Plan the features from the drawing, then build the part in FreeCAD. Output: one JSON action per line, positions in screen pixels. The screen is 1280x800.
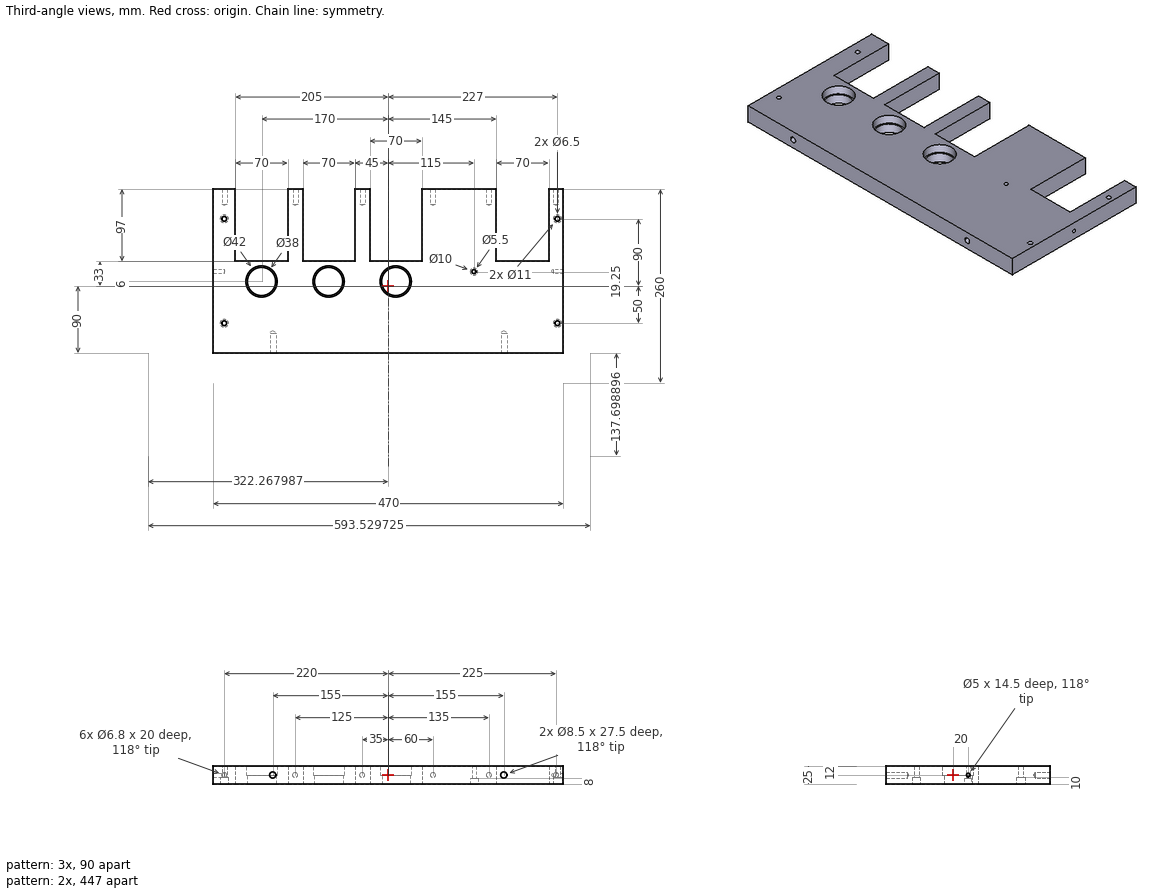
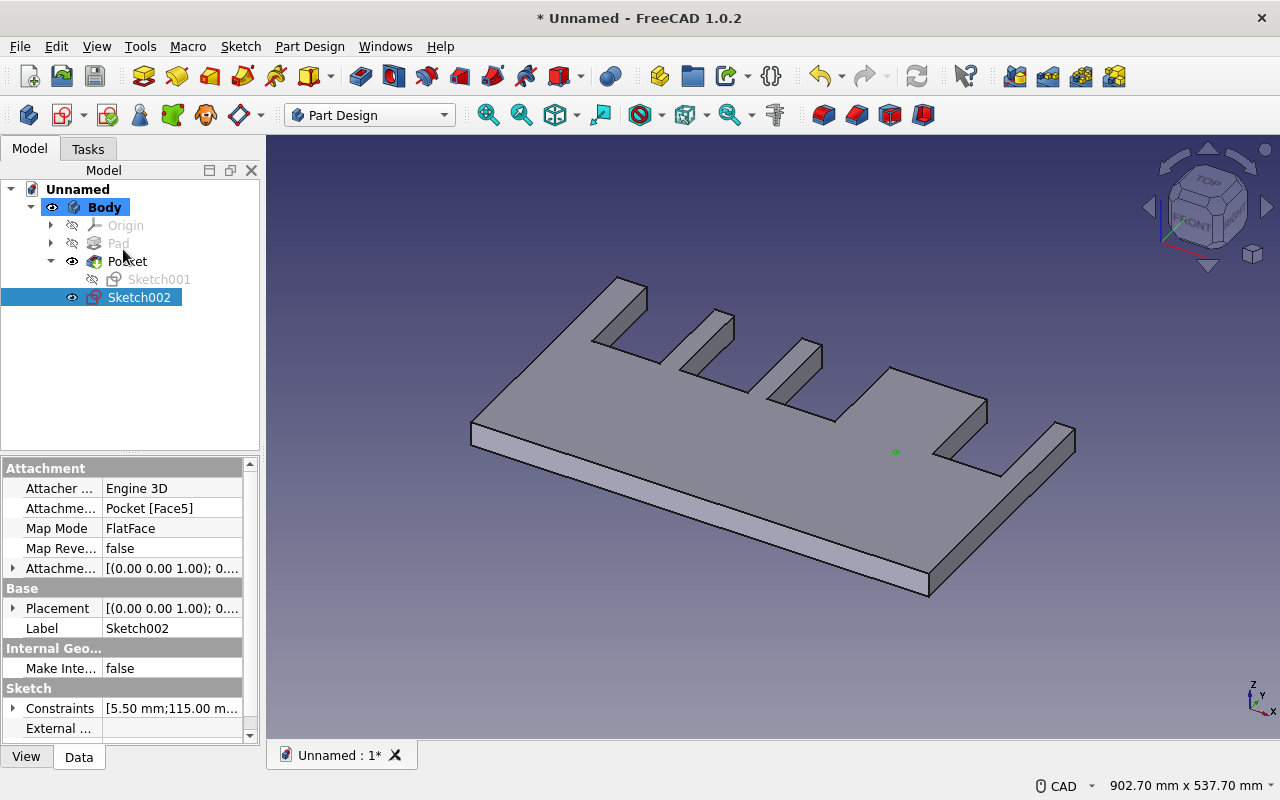
{"action": "left_click", "coordinate": [361, 76]}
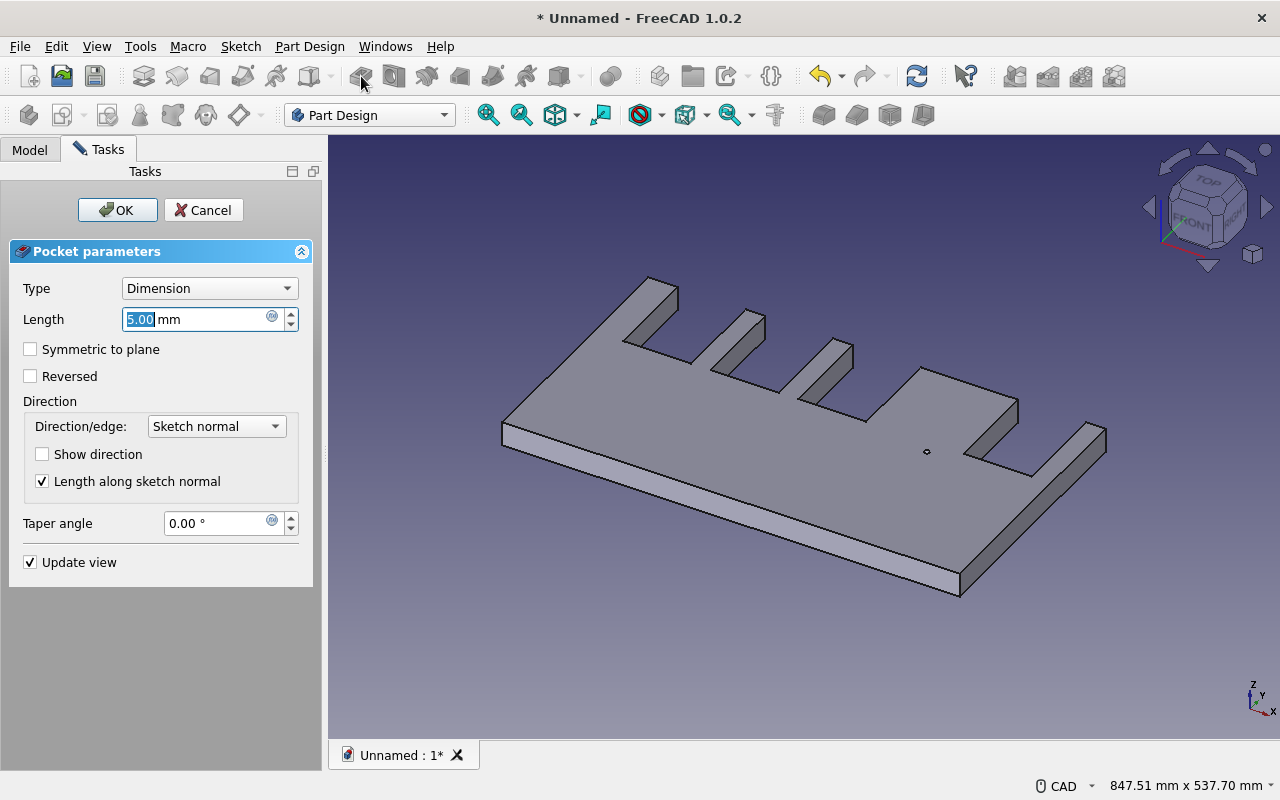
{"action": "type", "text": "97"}
{"action": "key", "text": "Tab"}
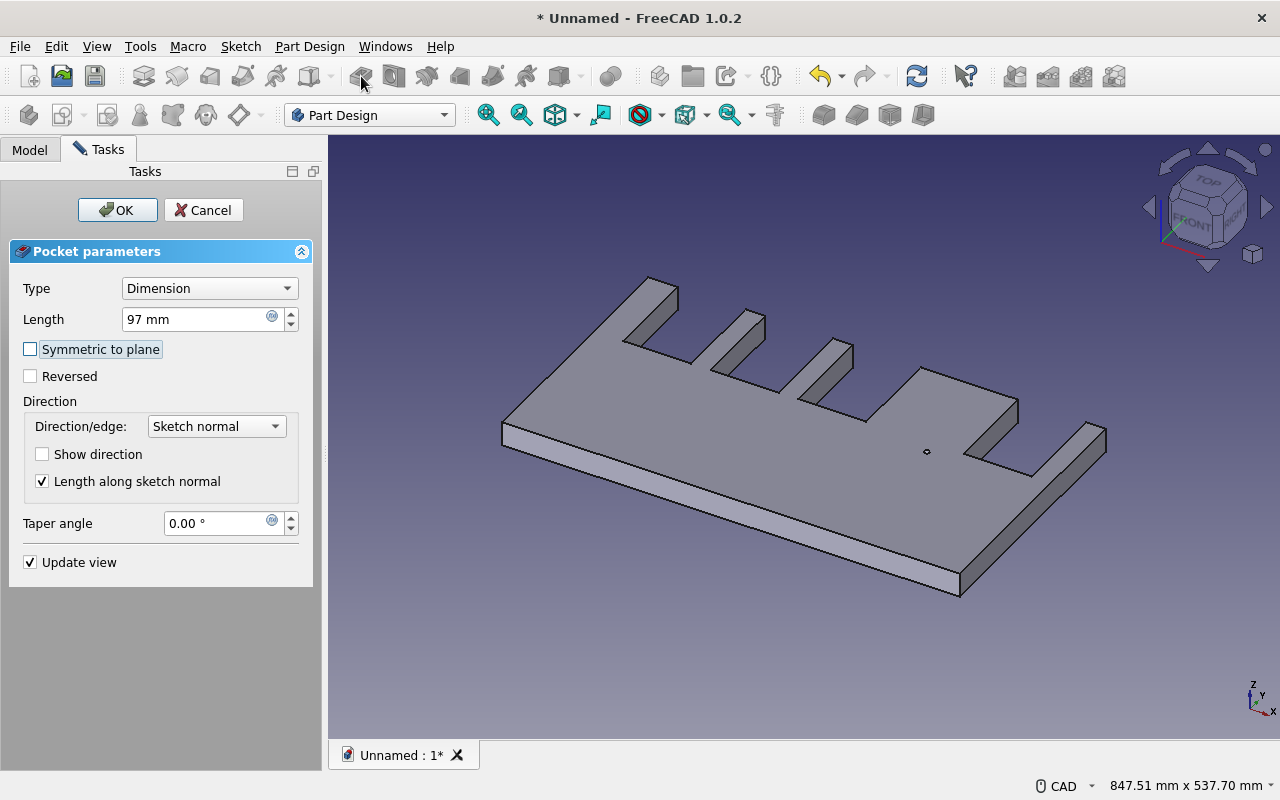
{"action": "left_click", "coordinate": [118, 210]}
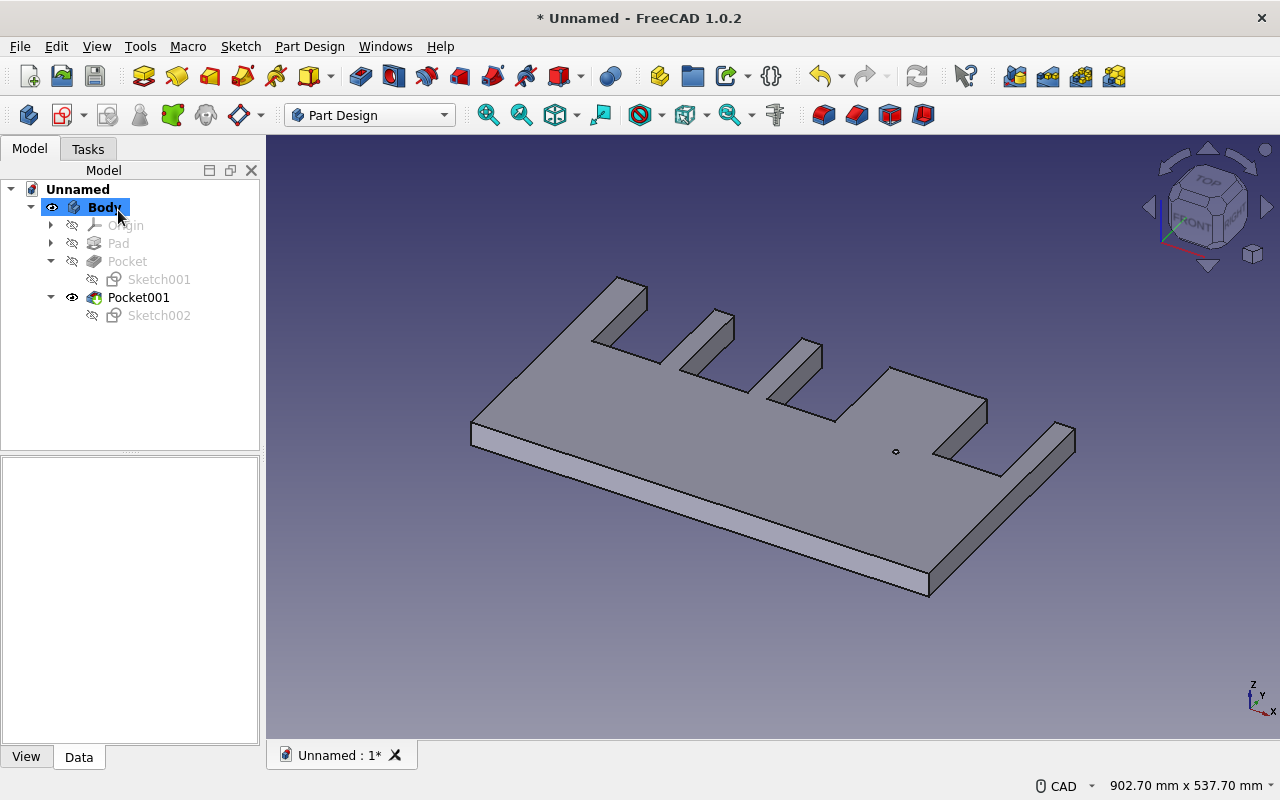
{"action": "key", "text": "5"}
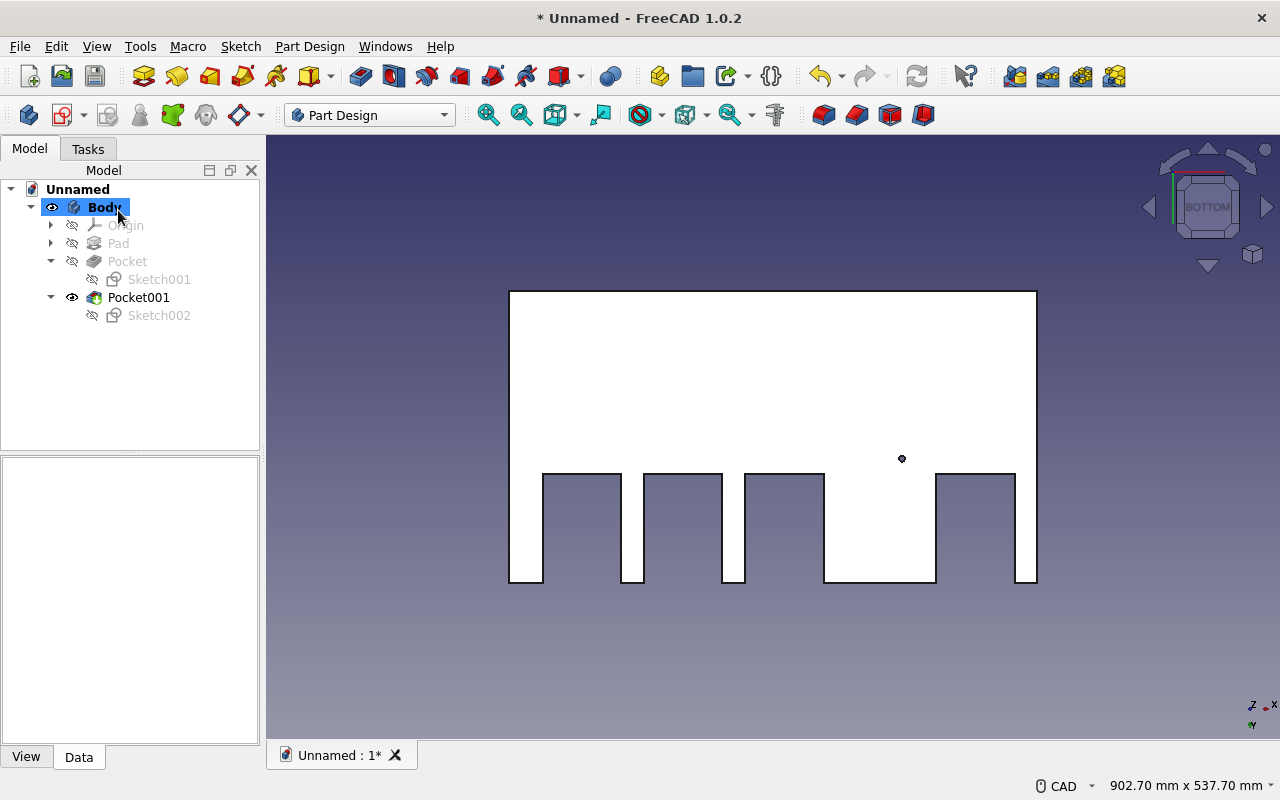
{"action": "left_click", "coordinate": [848, 394]}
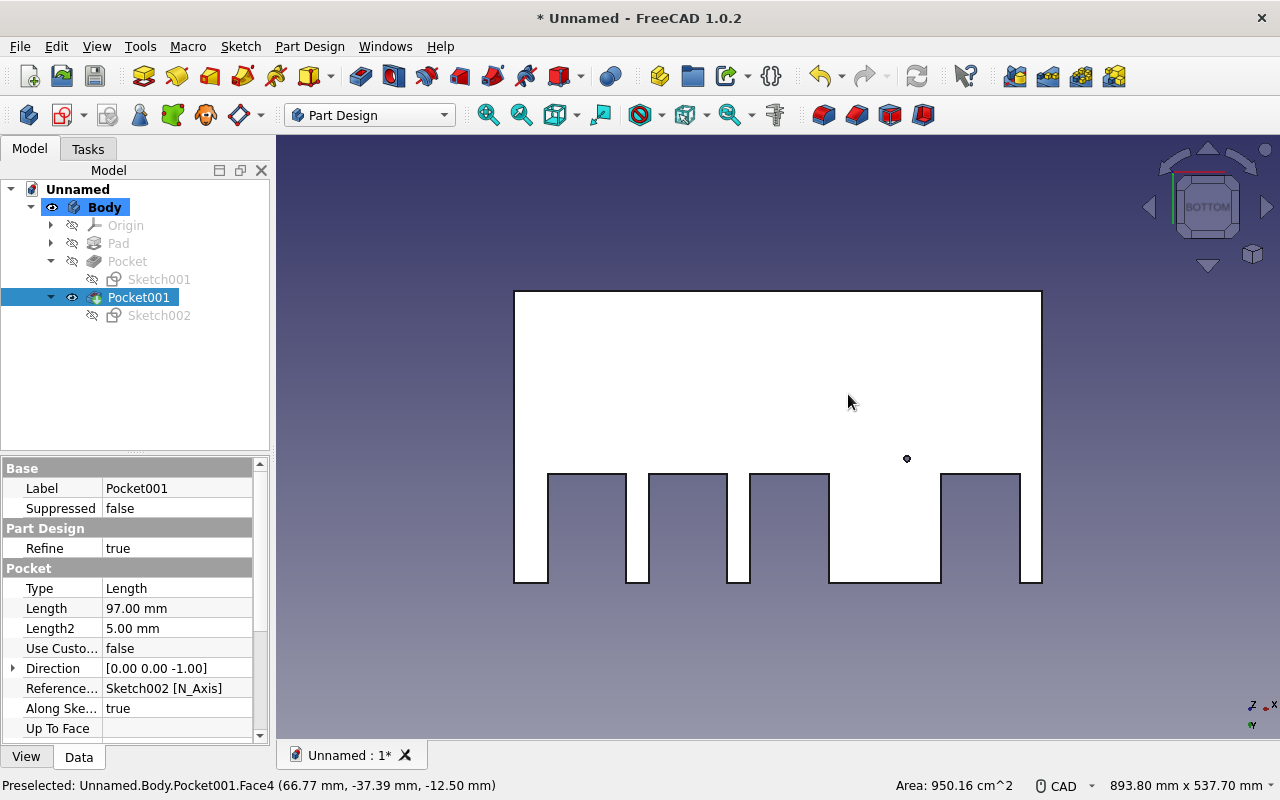
{"action": "left_click", "coordinate": [62, 116]}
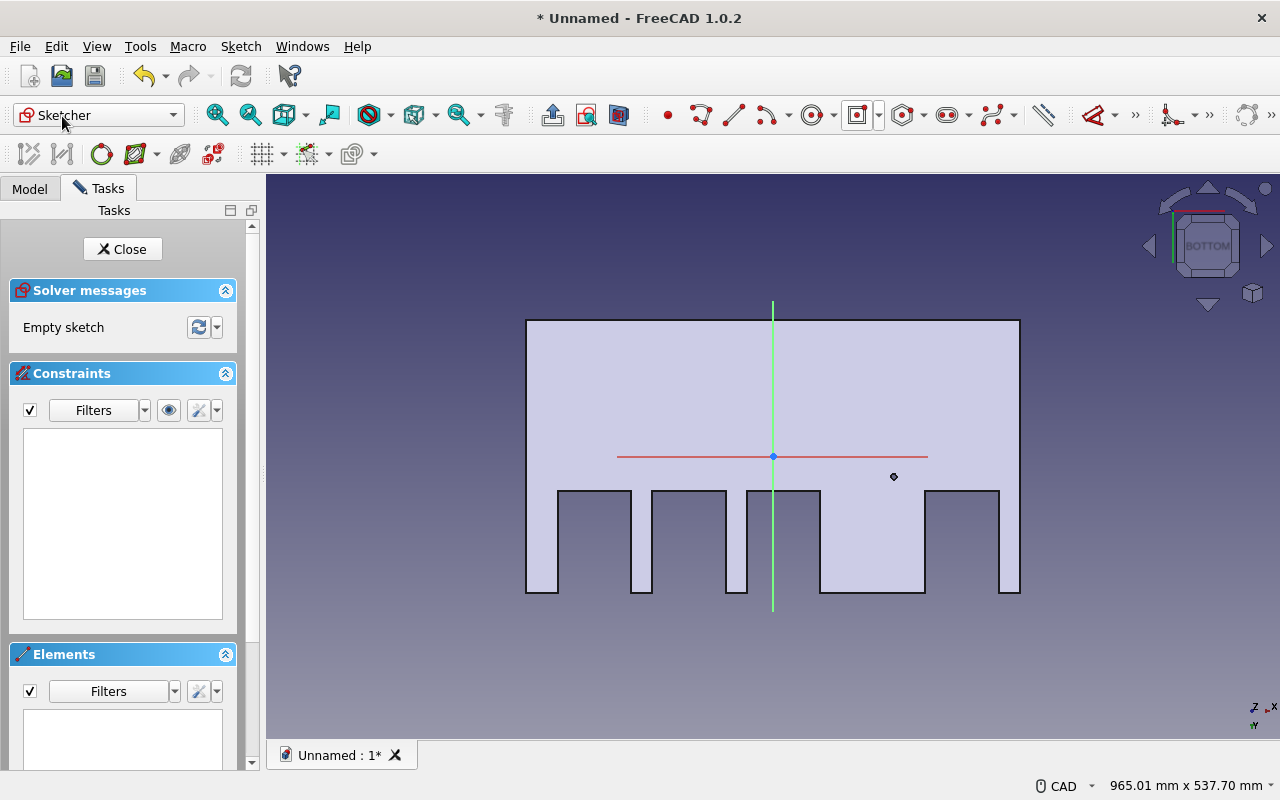
{"action": "scroll", "coordinate": [904, 478], "scroll_direction": "up", "scroll_amount": 15}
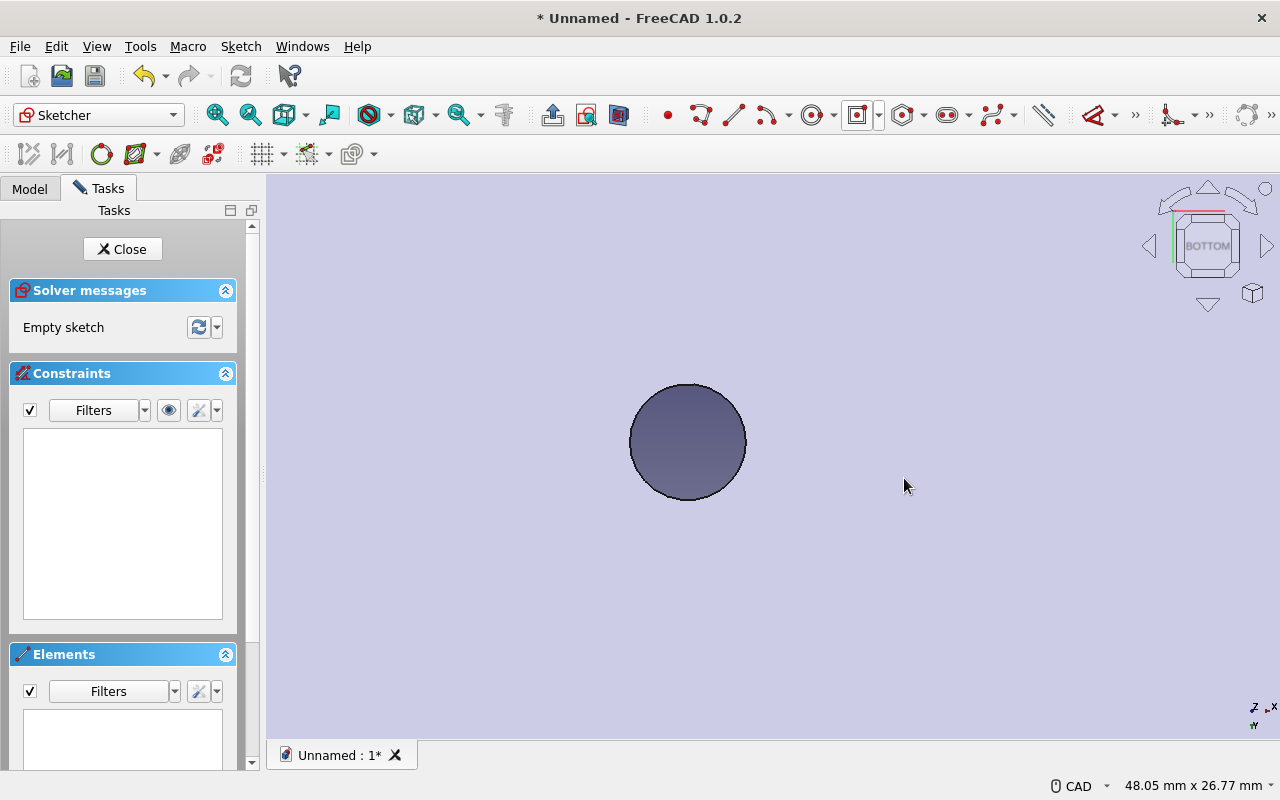
{"action": "scroll", "coordinate": [668, 425], "scroll_direction": "up", "scroll_amount": 3}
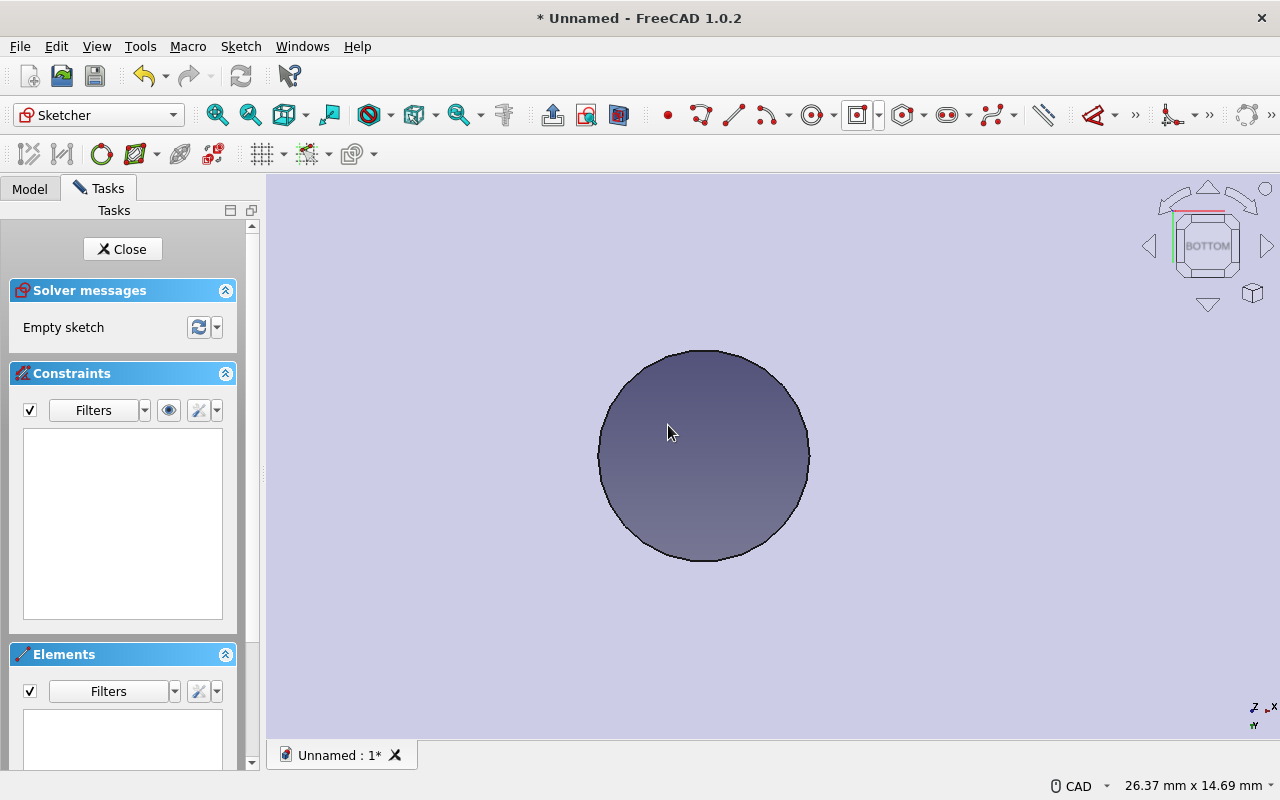
{"action": "left_click", "coordinate": [812, 116]}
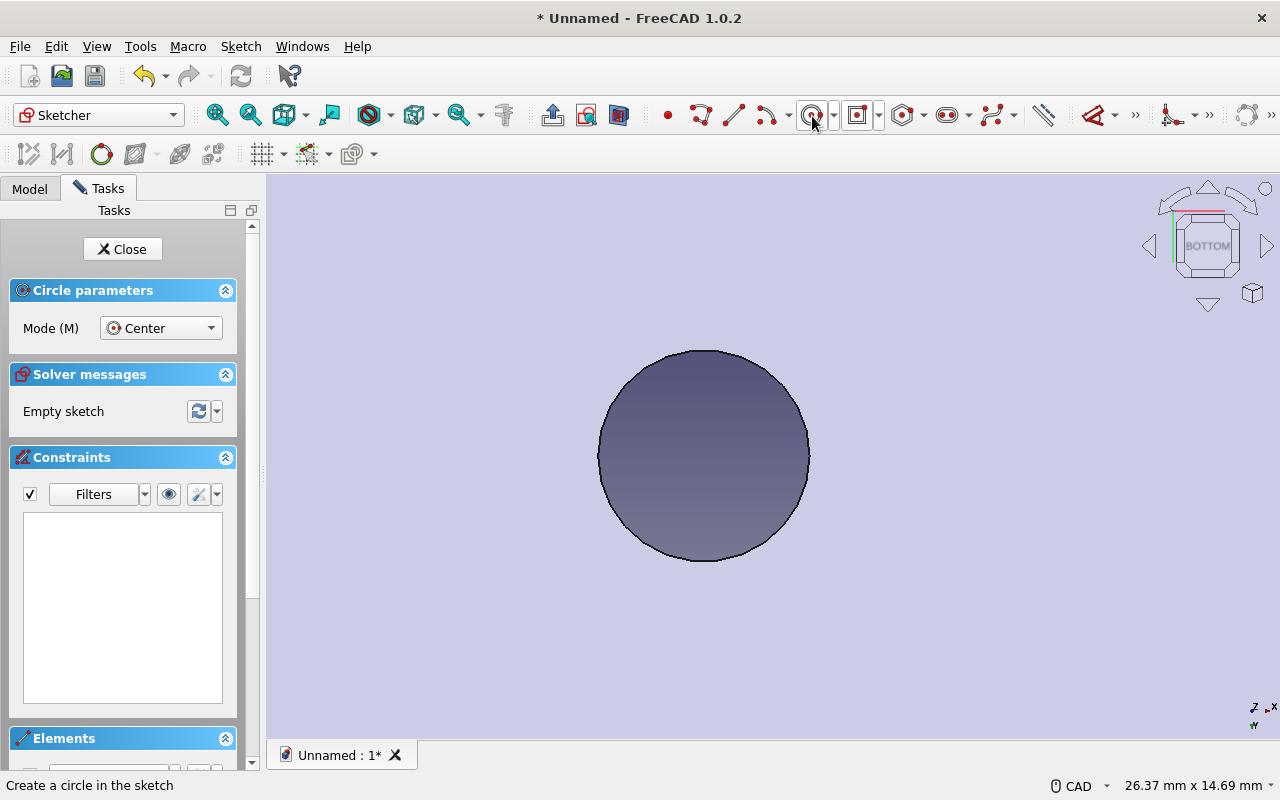
{"action": "left_click", "coordinate": [704, 456]}
{"action": "mouse_move", "coordinate": [840, 320]}